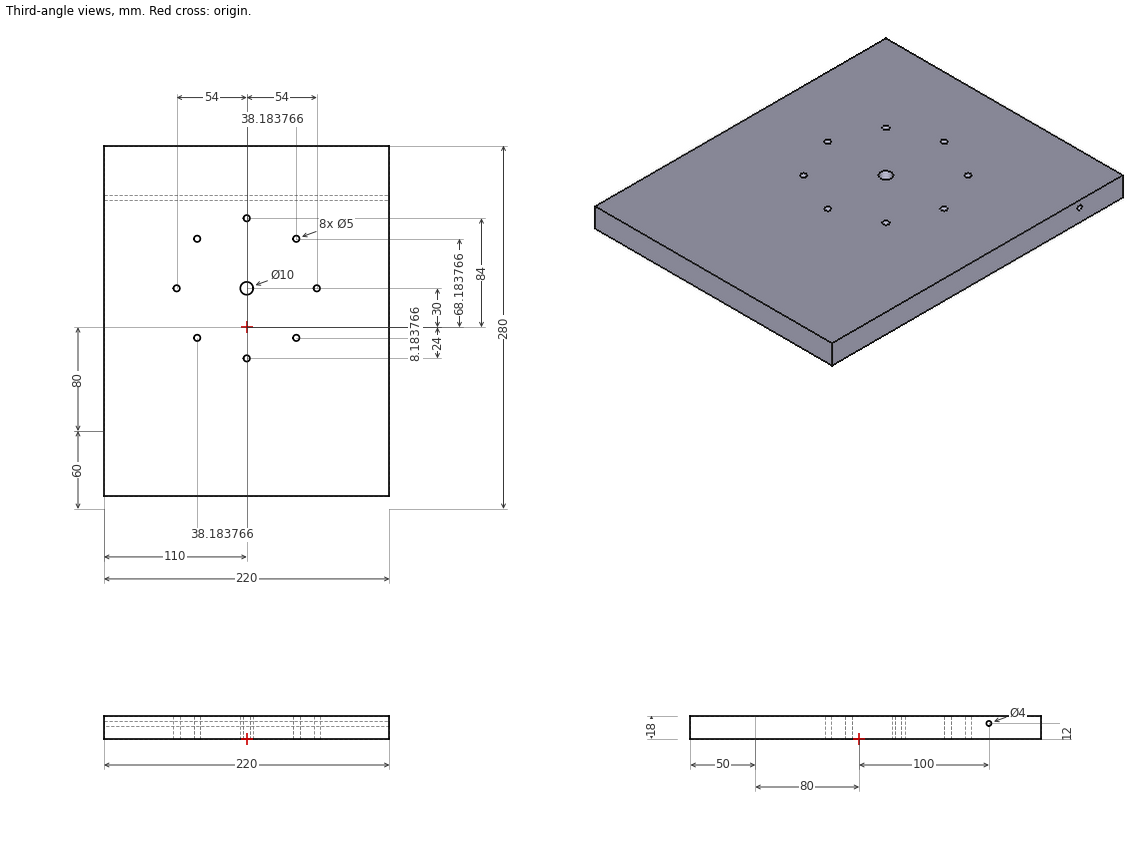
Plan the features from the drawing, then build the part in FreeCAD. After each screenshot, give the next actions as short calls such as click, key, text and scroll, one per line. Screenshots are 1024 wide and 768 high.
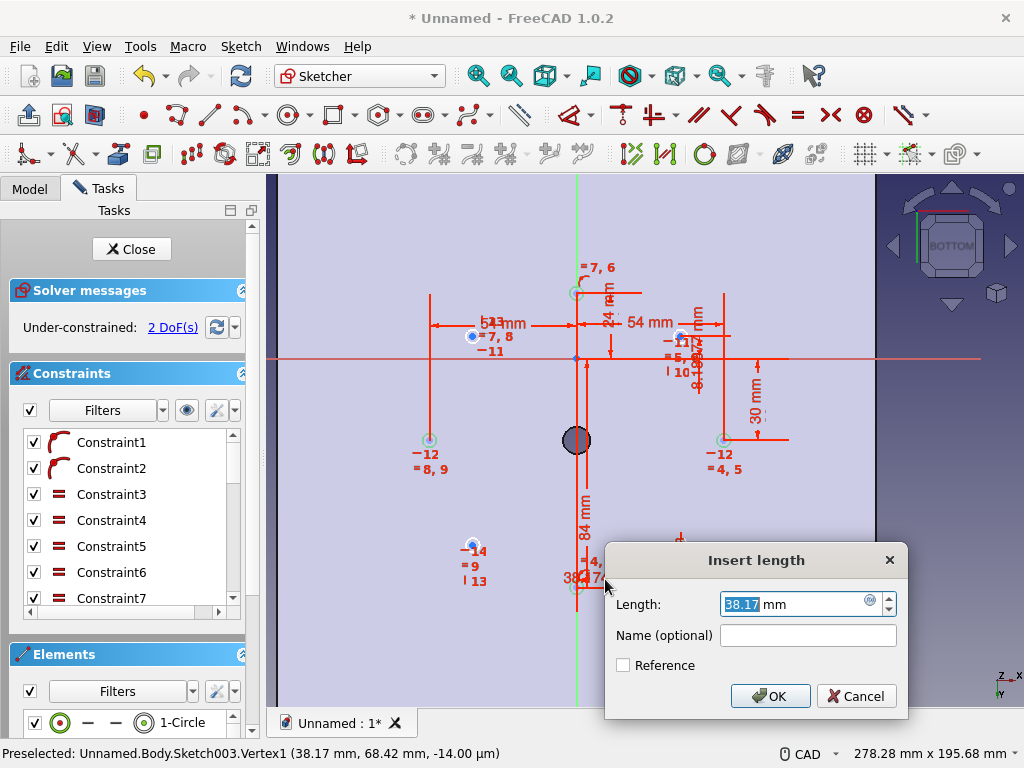
text(38.183766)
key(Return)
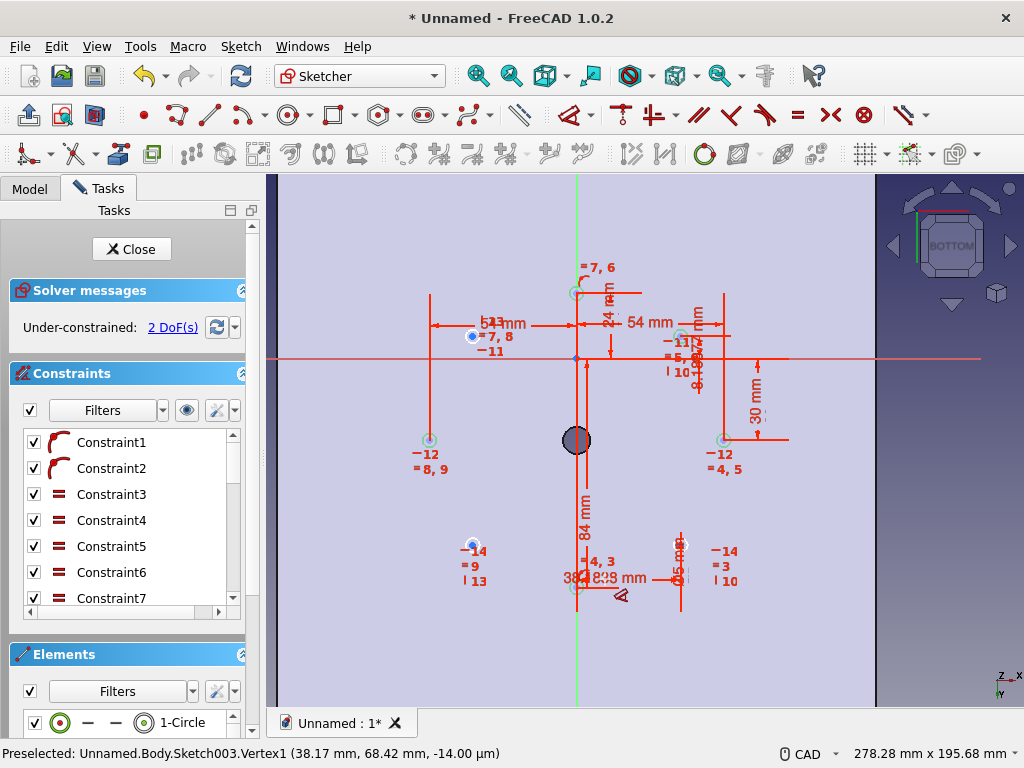
click(681, 545)
click(715, 495)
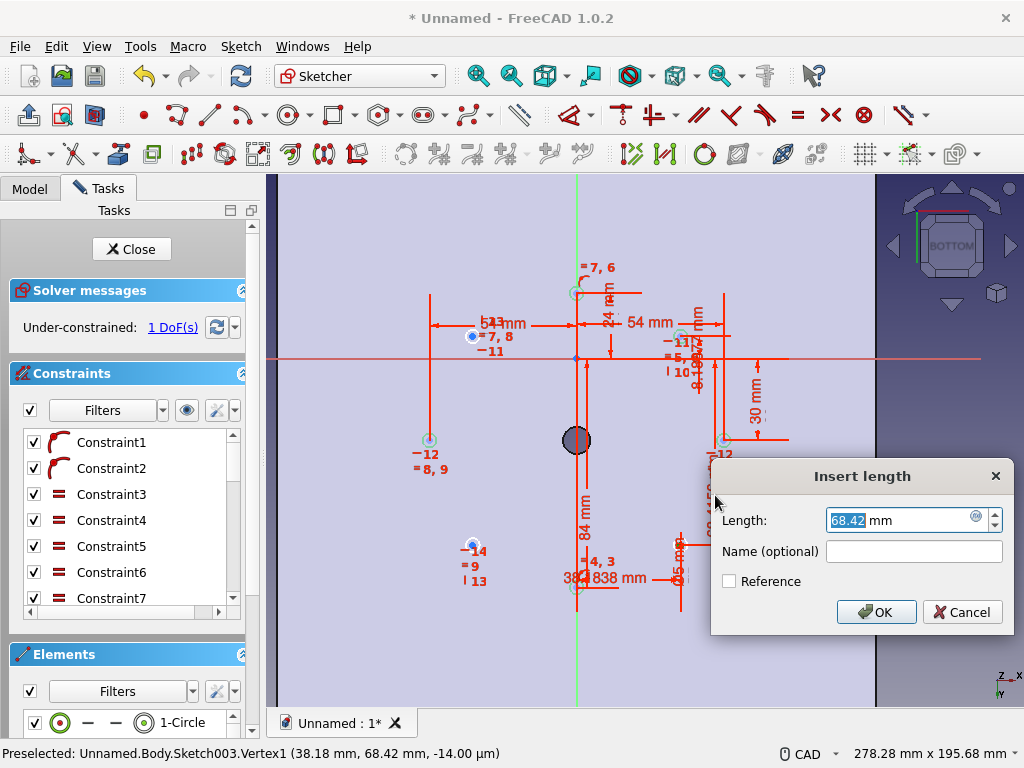
text(68.183766)
key(Return)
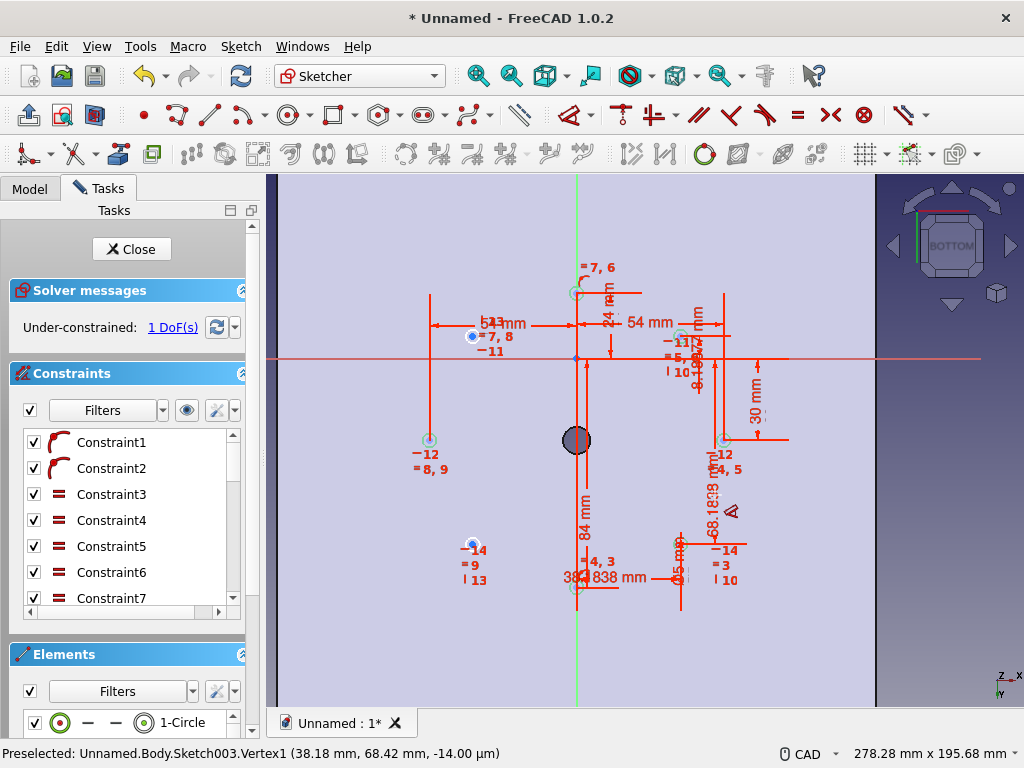
click(473, 336)
click(525, 302)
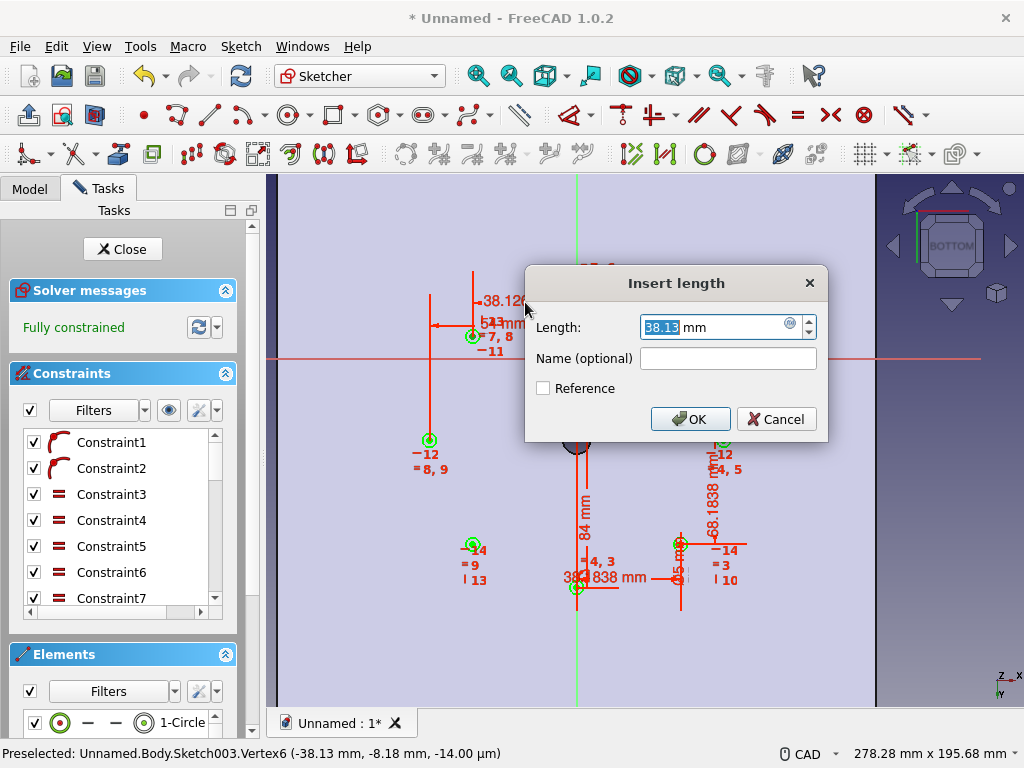
text(38.183766)
key(Return)
key(Escape)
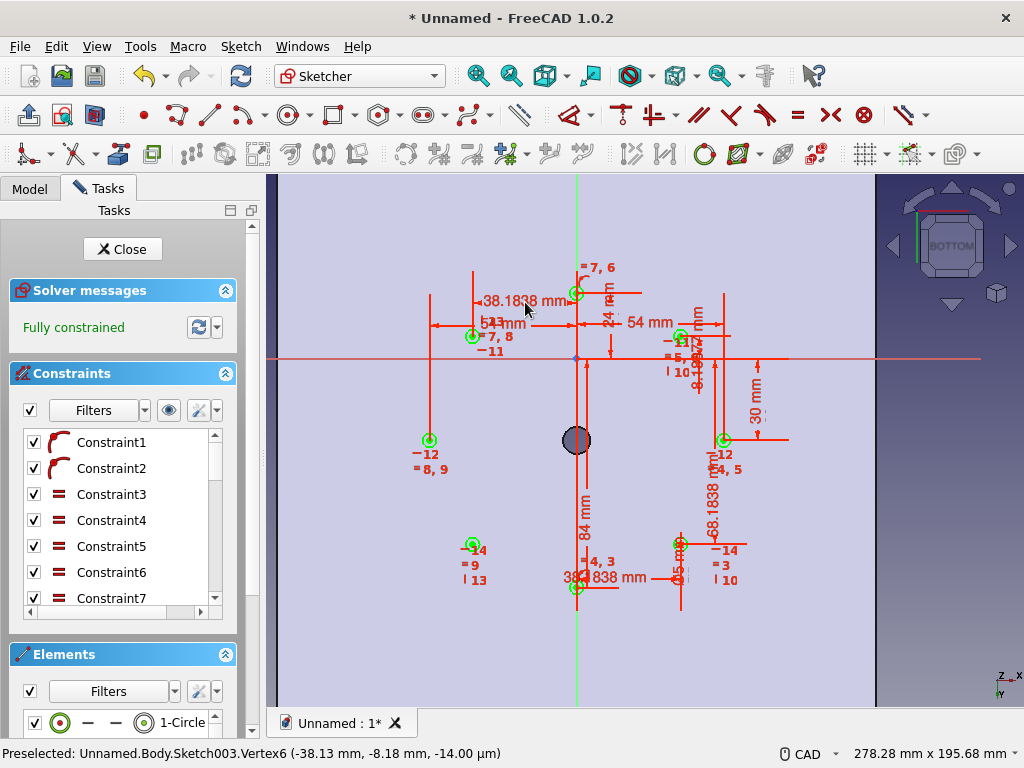
click(123, 249)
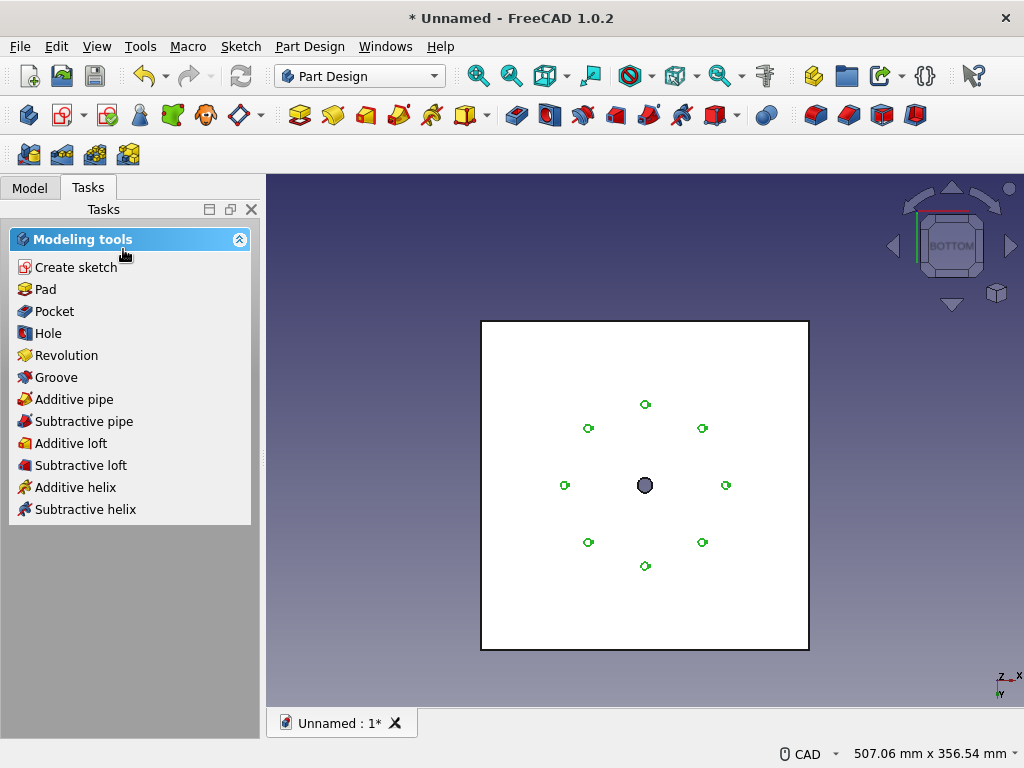
click(517, 116)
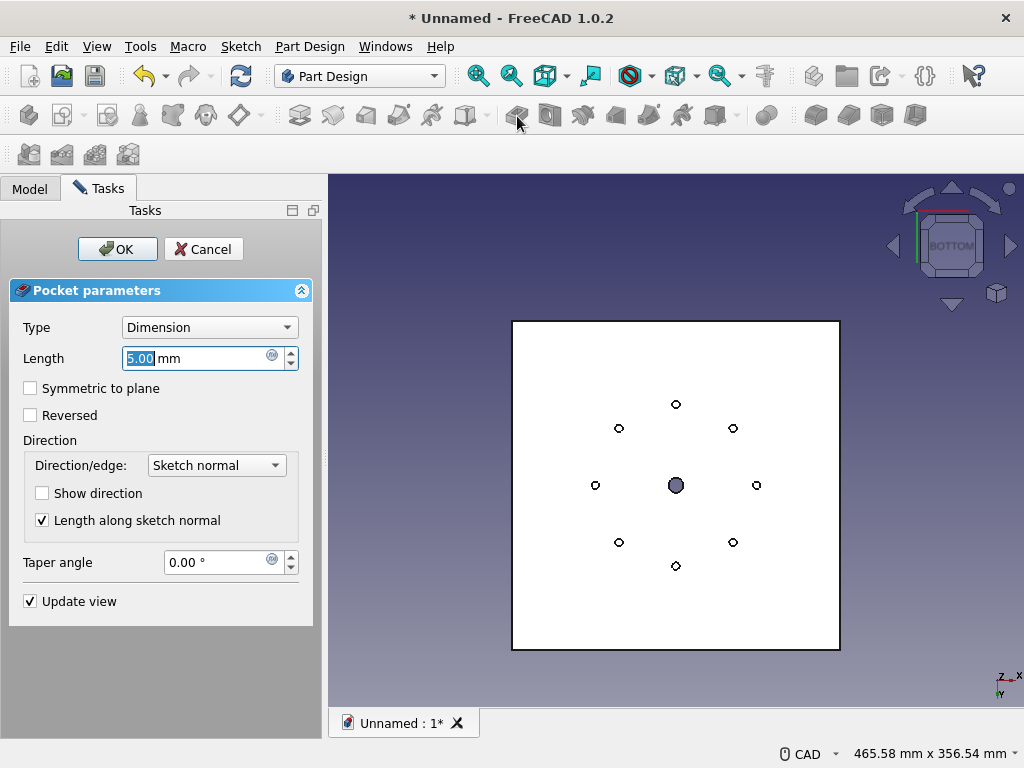
click(210, 328)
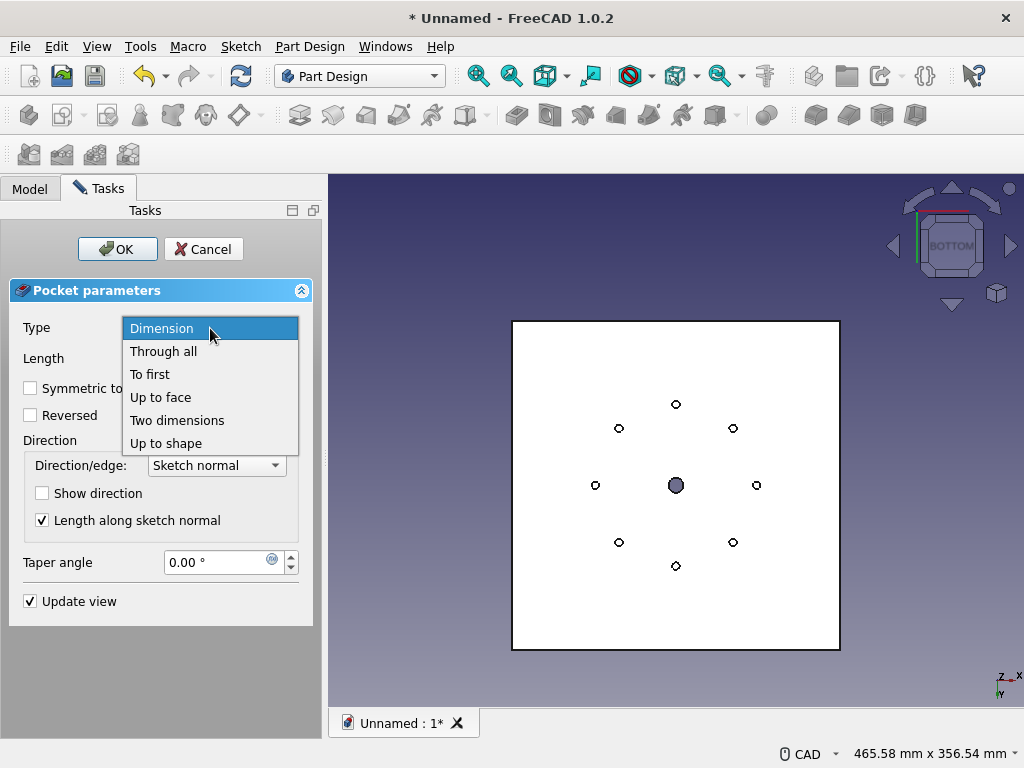
click(208, 352)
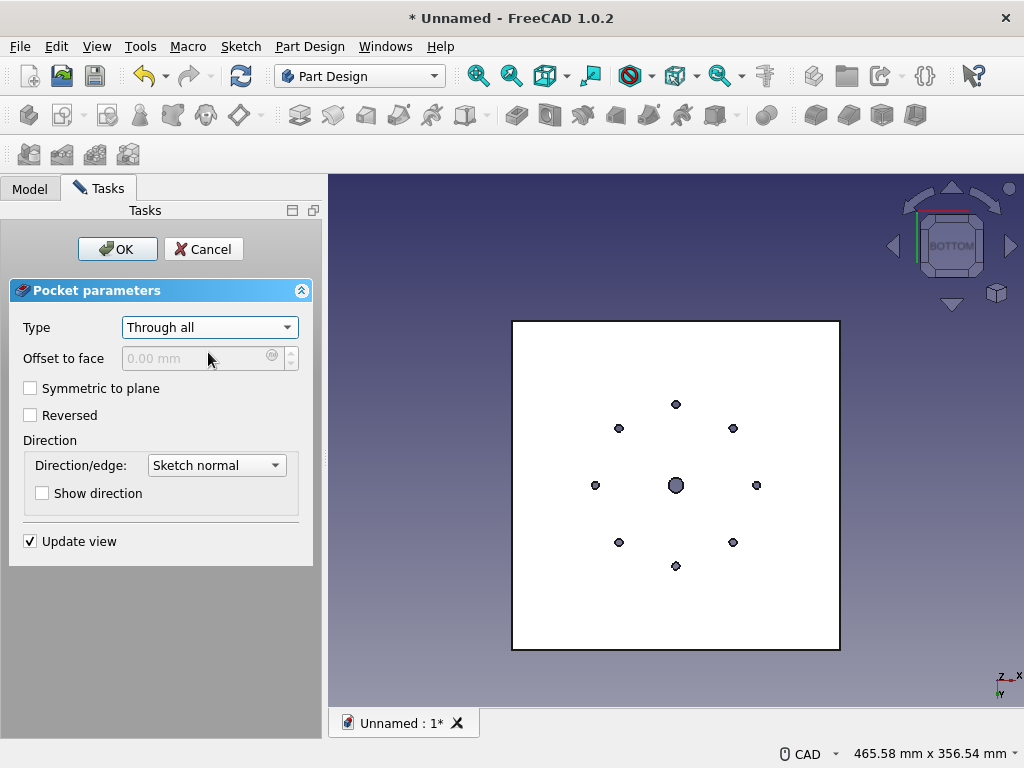
click(118, 249)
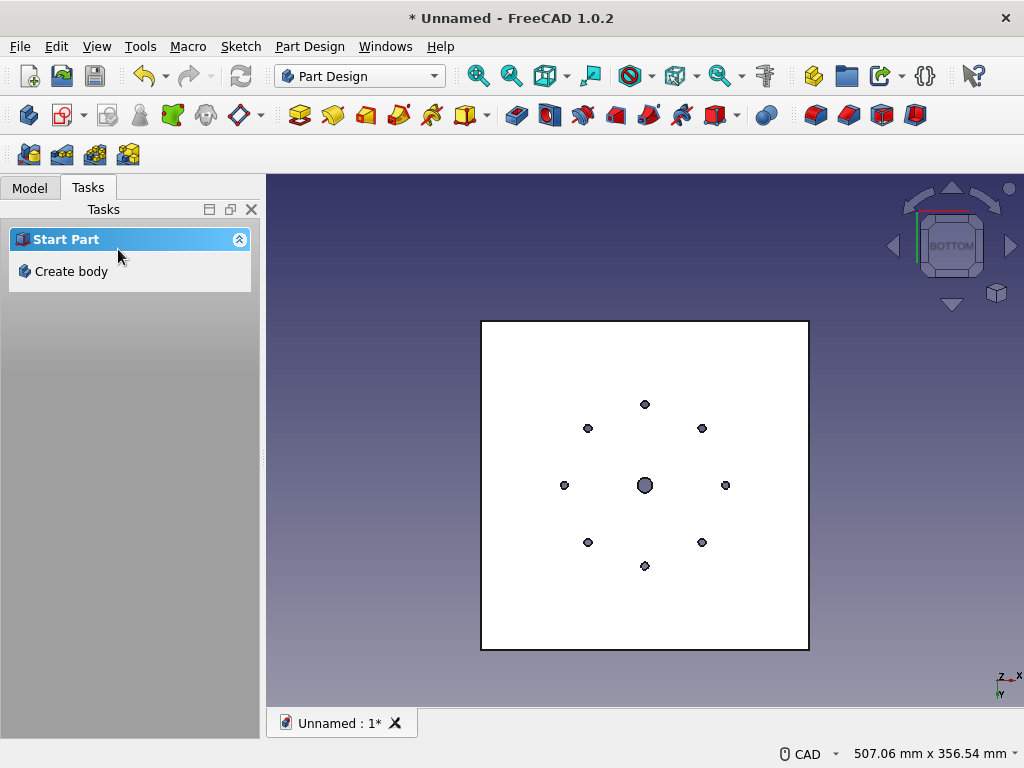
key(6)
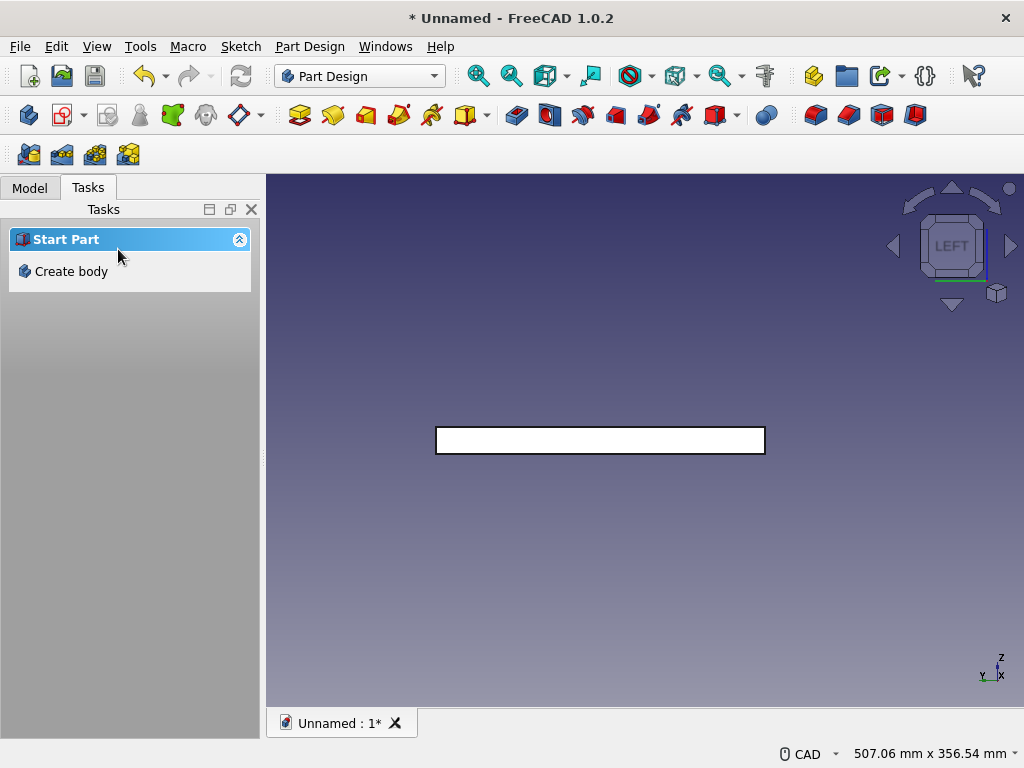
click(479, 76)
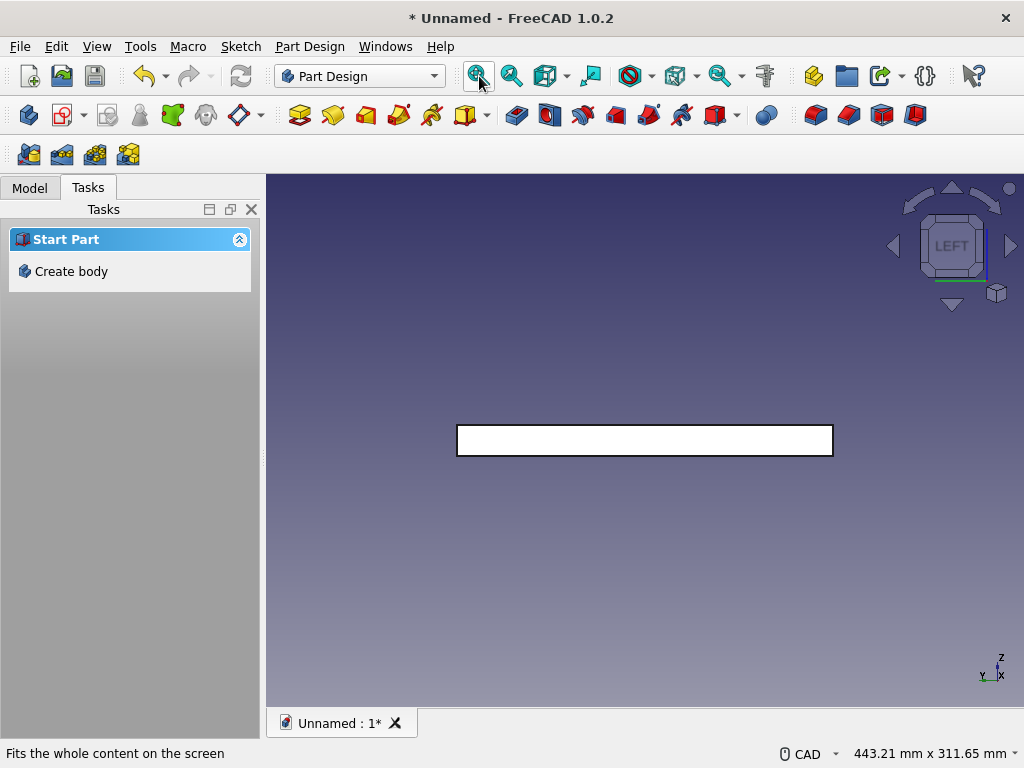
click(484, 439)